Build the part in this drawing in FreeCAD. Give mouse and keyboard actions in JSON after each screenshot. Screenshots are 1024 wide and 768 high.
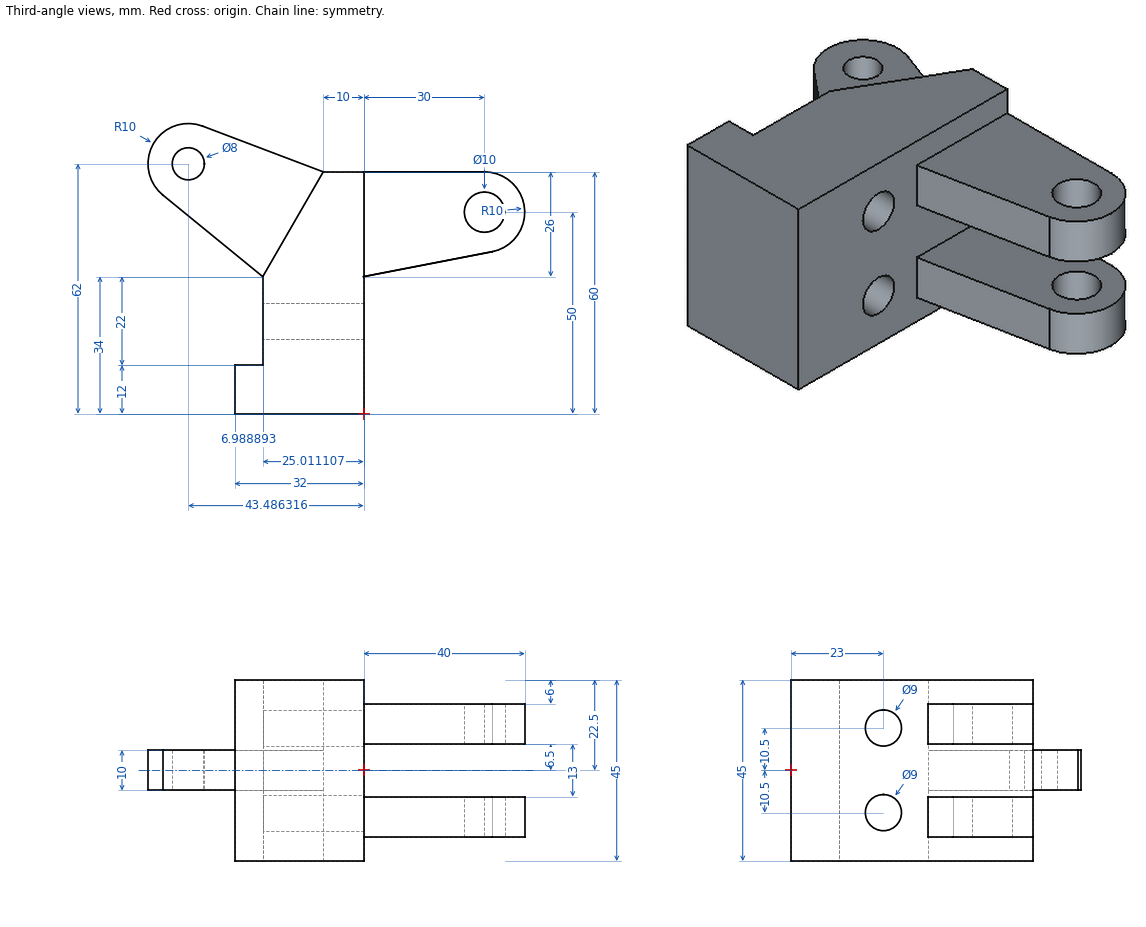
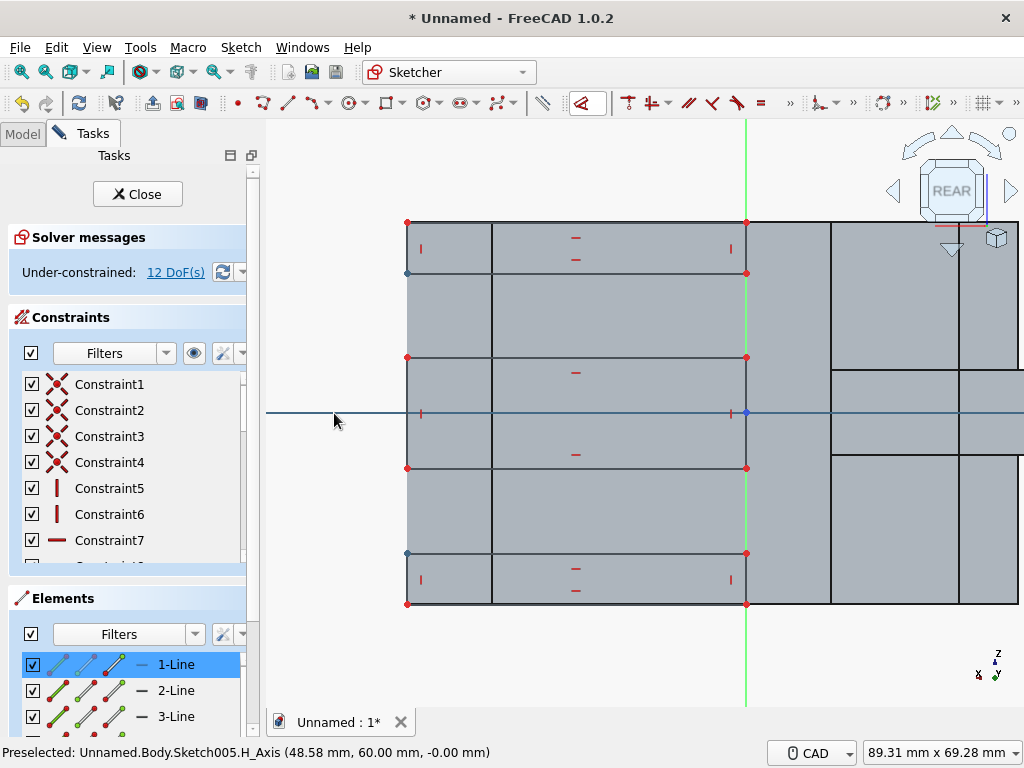
{"action": "key", "text": "s"}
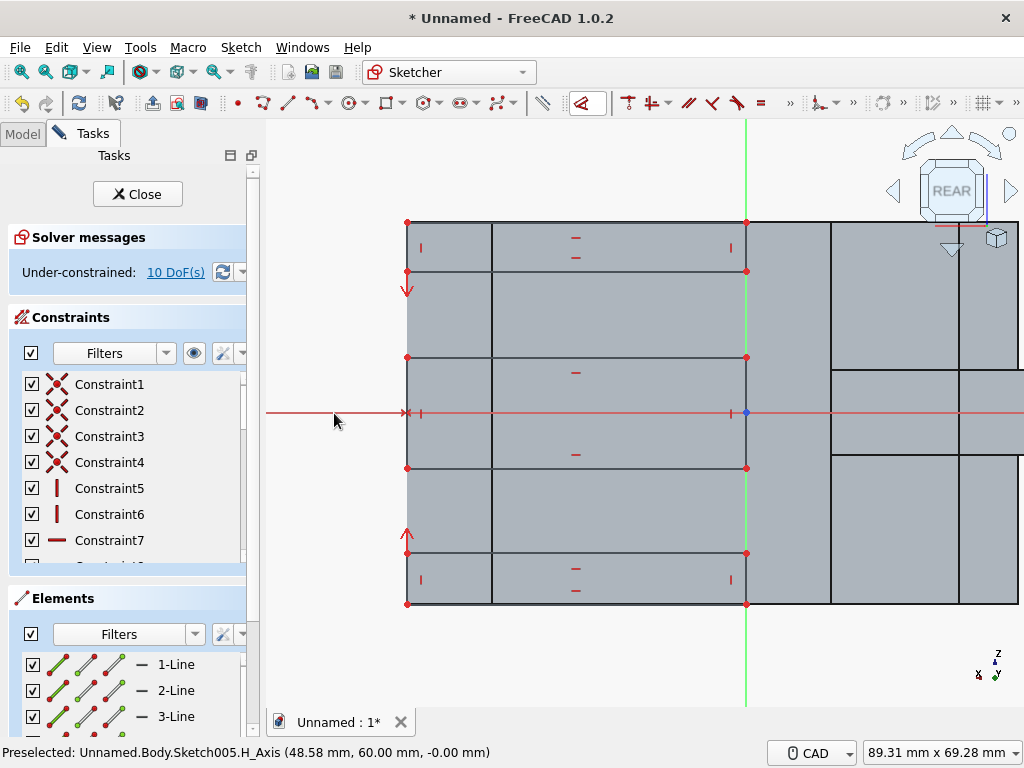
{"action": "left_click", "coordinate": [746, 223]}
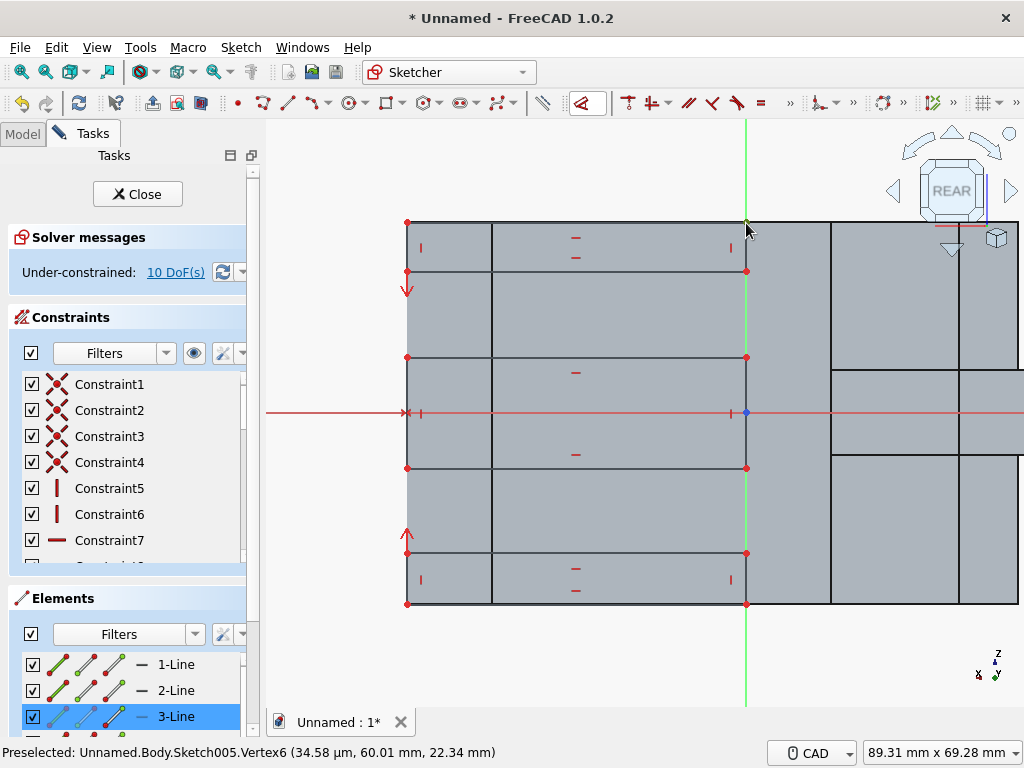
{"action": "left_click", "coordinate": [746, 605]}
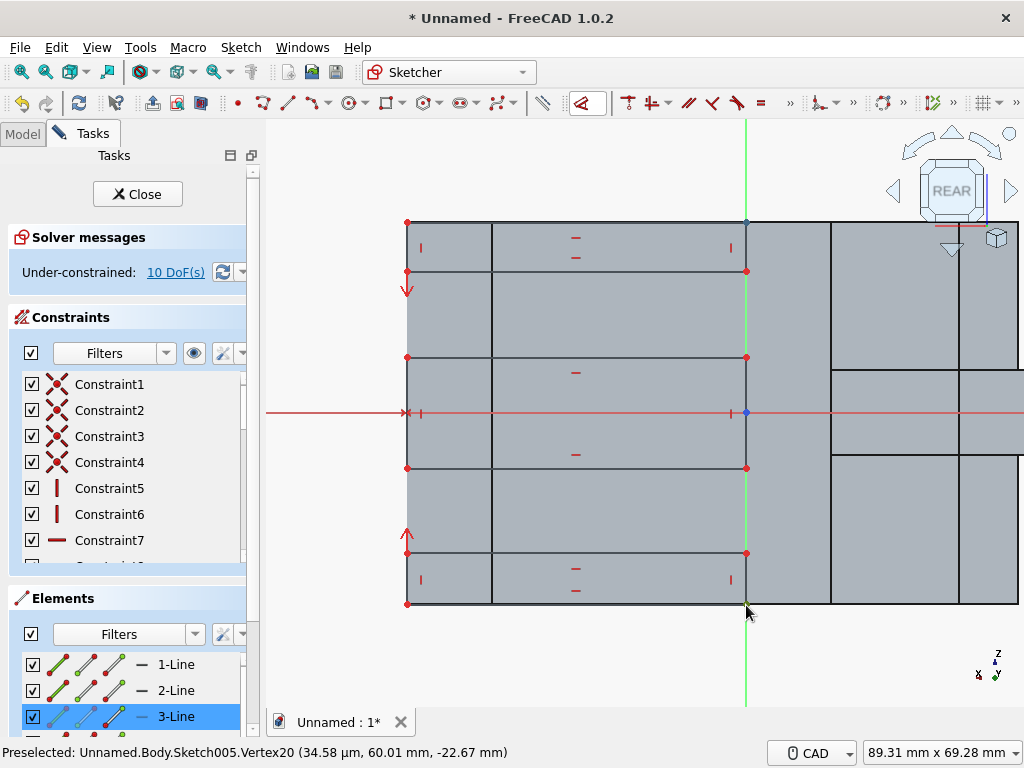
{"action": "left_click", "coordinate": [334, 413]}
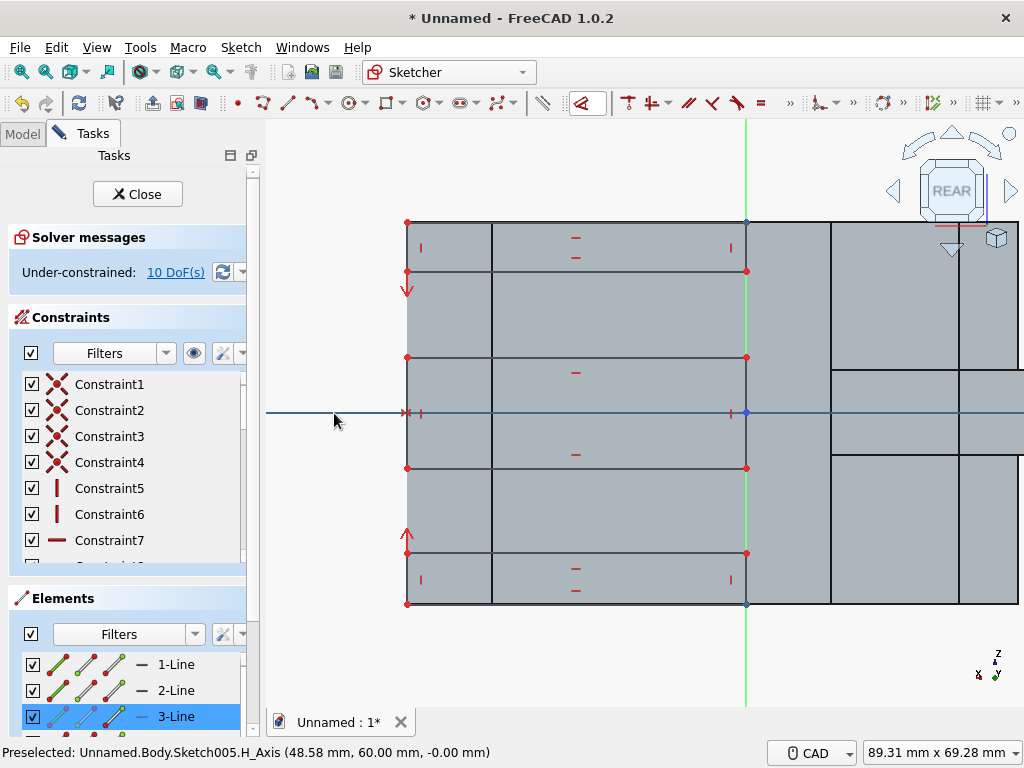
{"action": "key", "text": "s"}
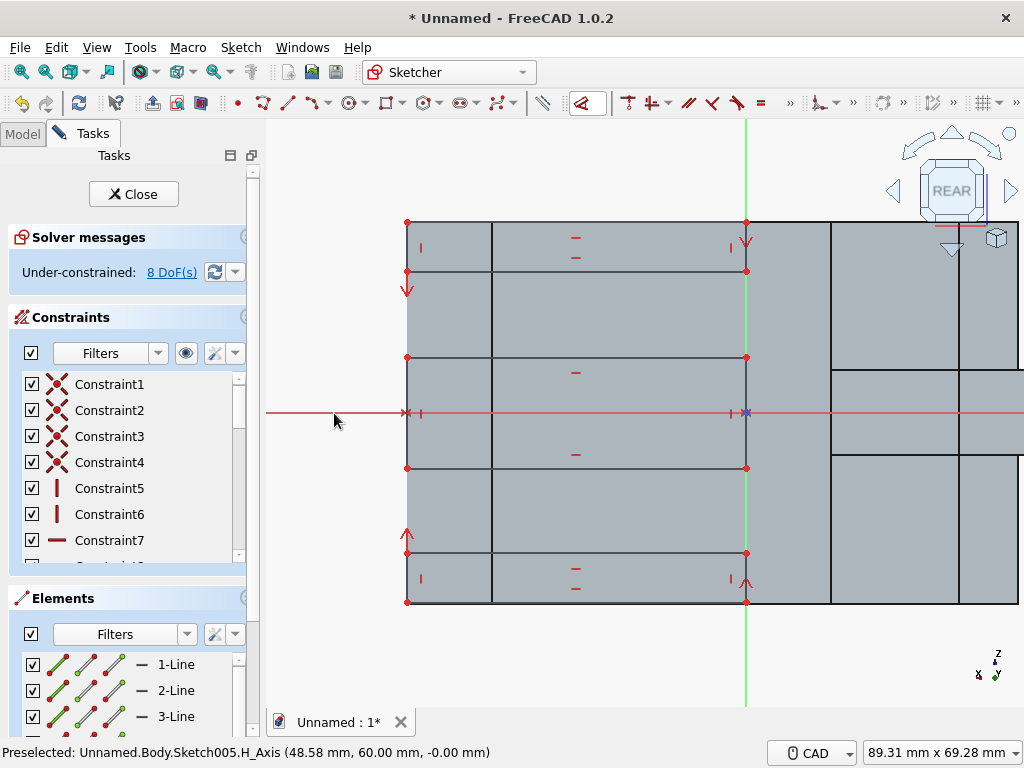
{"action": "left_click", "coordinate": [746, 272]}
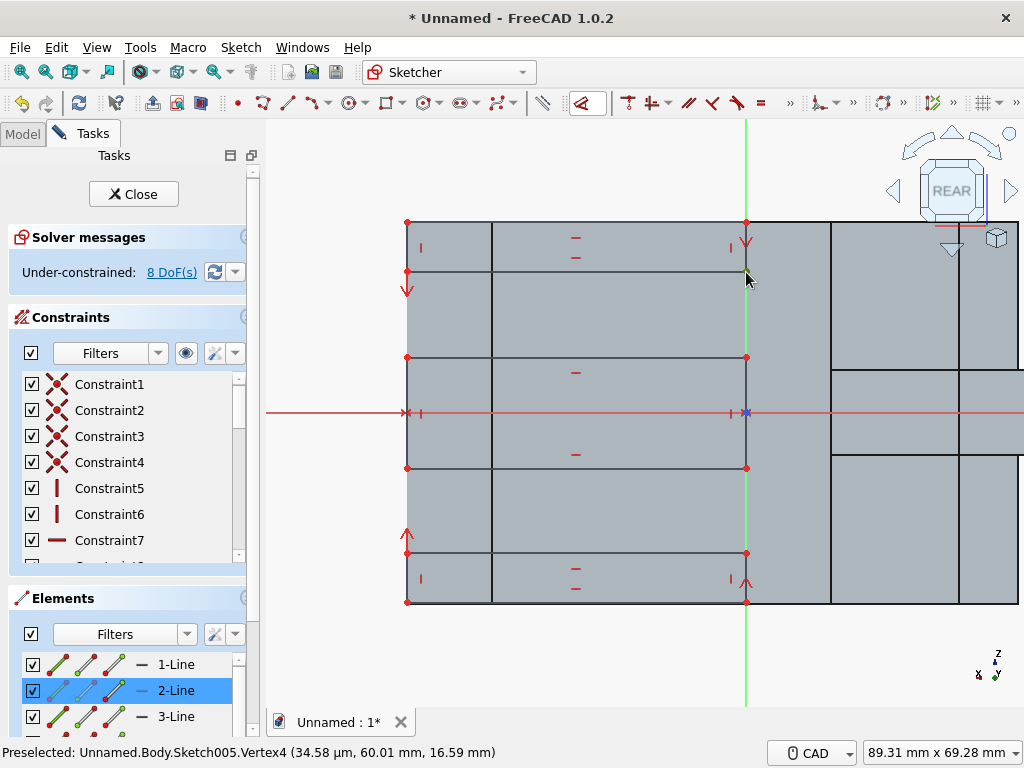
{"action": "left_click", "coordinate": [746, 641]}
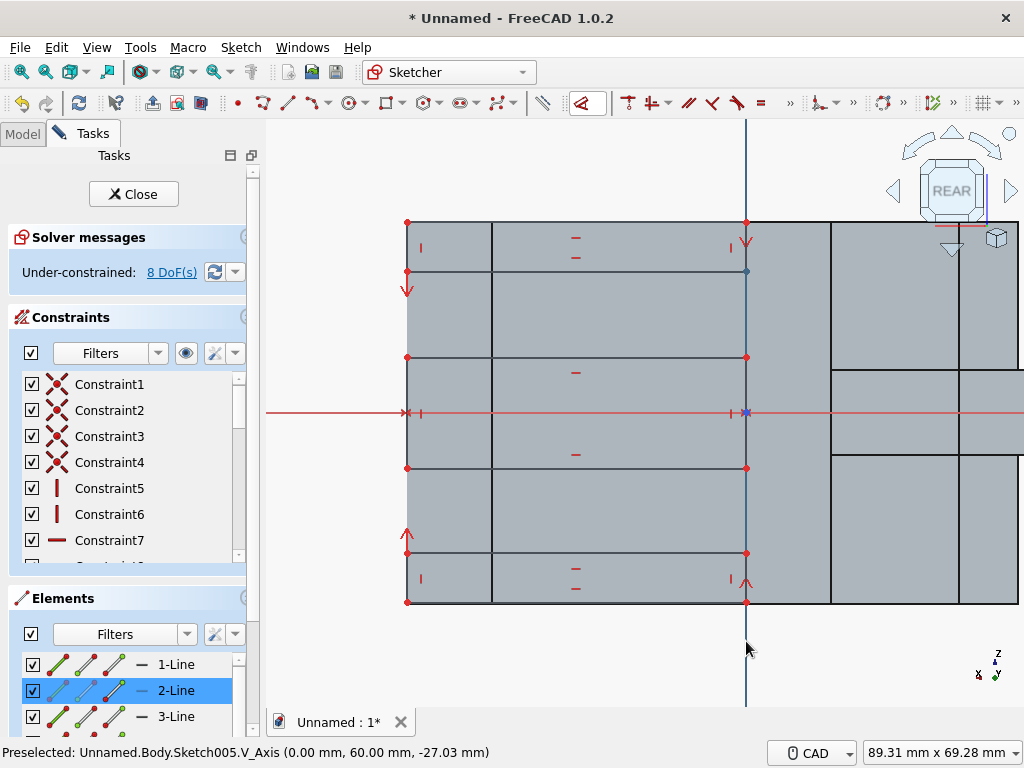
{"action": "left_click", "coordinate": [628, 104]}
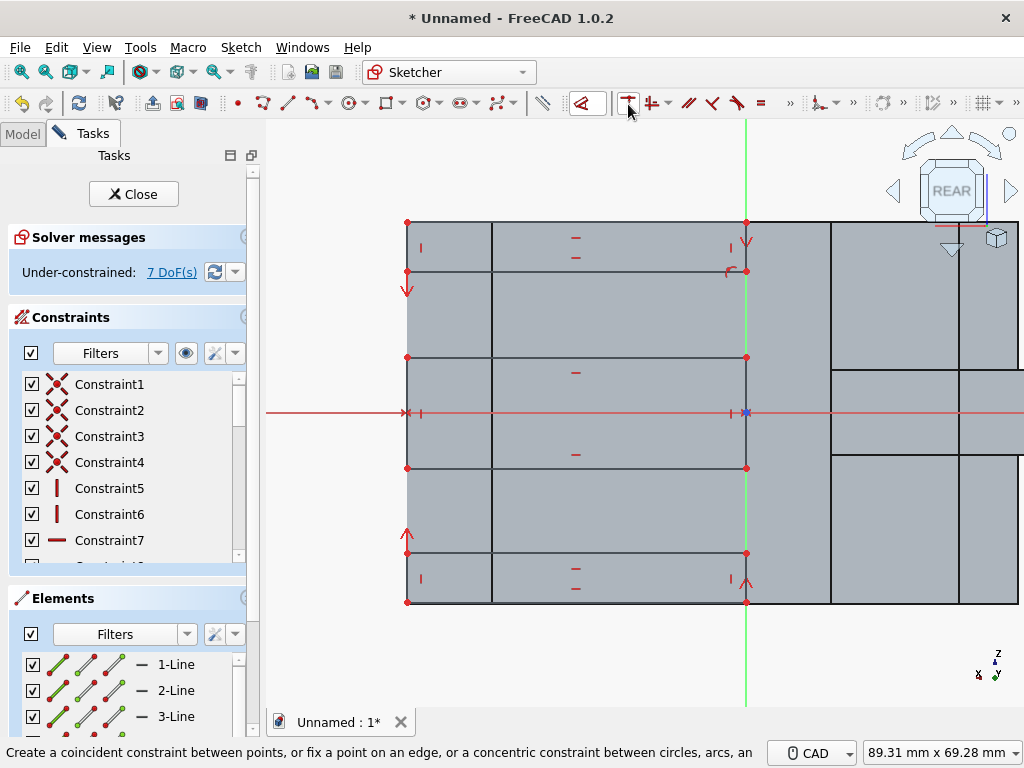
{"action": "left_click", "coordinate": [746, 469]}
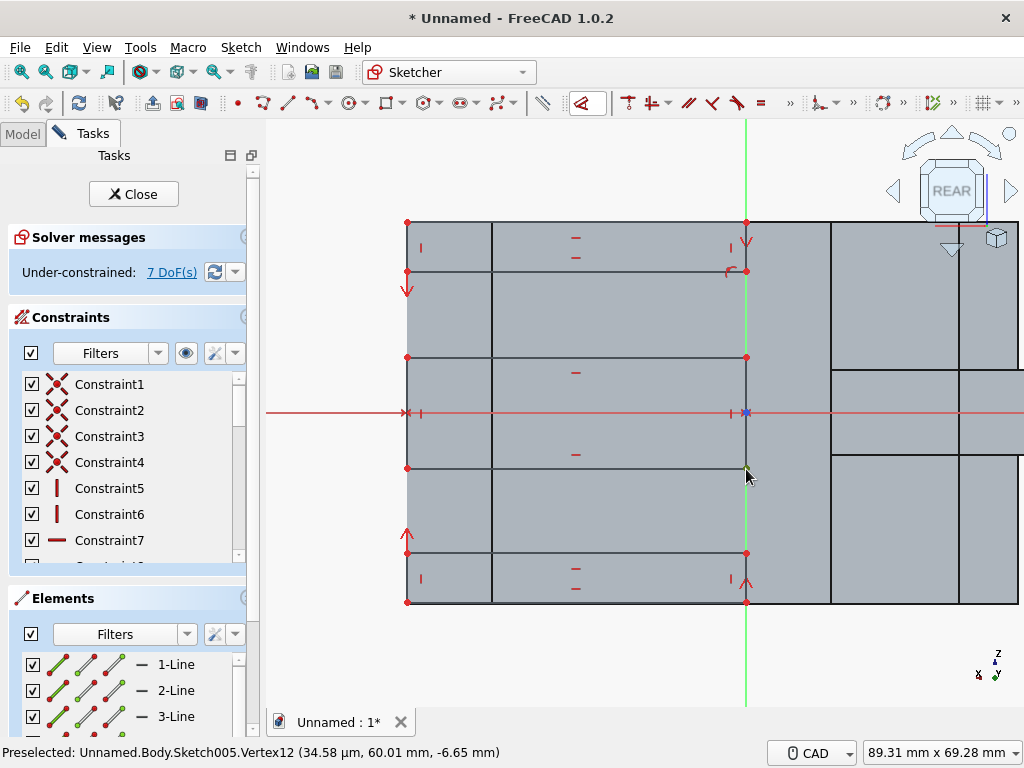
{"action": "left_click", "coordinate": [746, 641]}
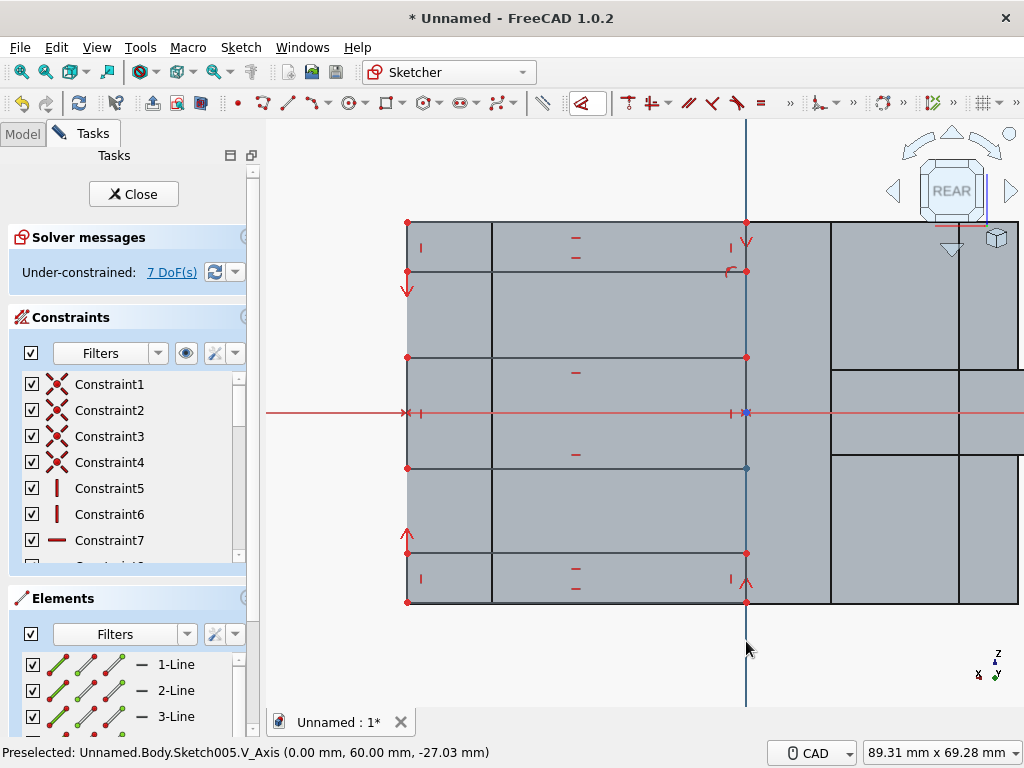
{"action": "left_click", "coordinate": [628, 104]}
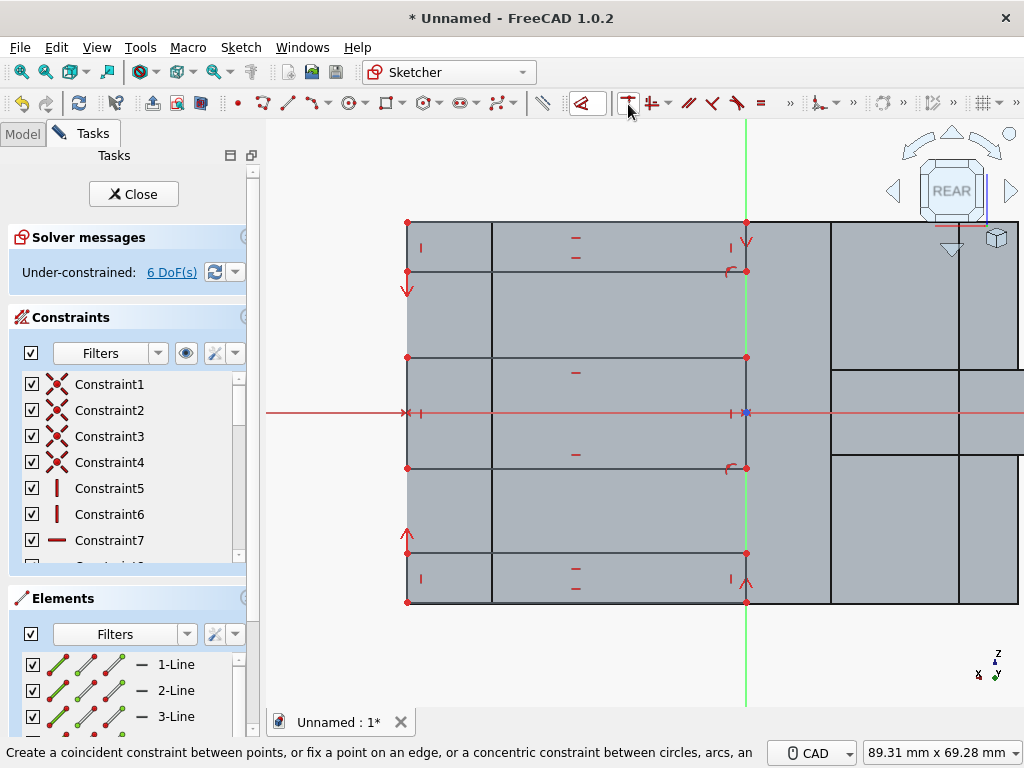
{"action": "left_click", "coordinate": [407, 237]}